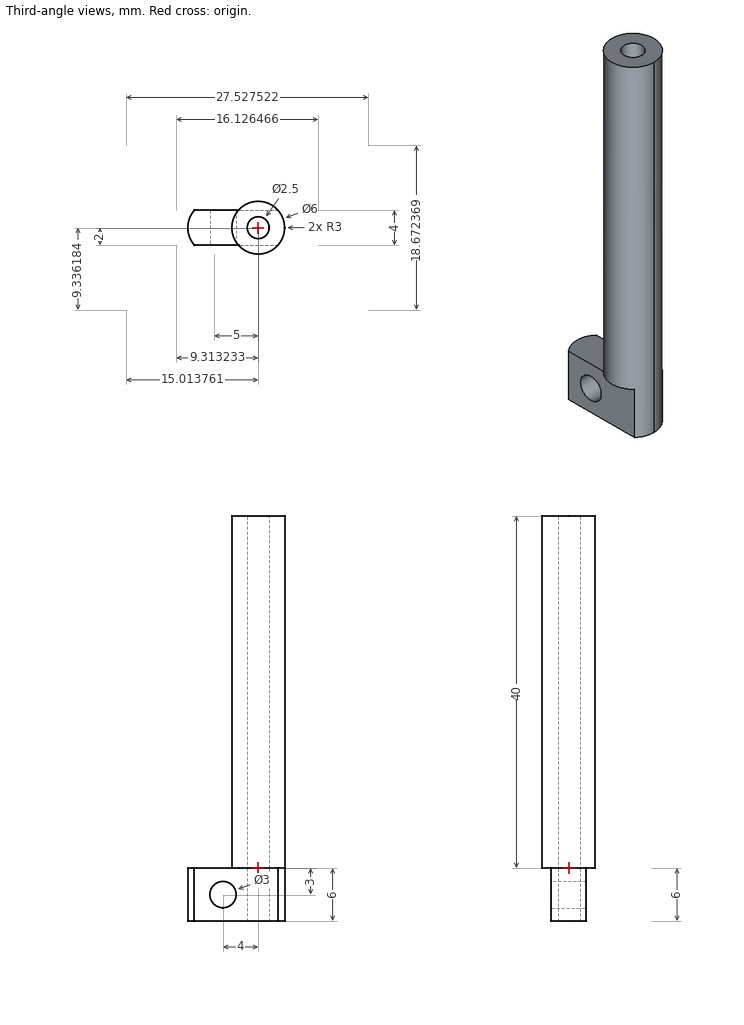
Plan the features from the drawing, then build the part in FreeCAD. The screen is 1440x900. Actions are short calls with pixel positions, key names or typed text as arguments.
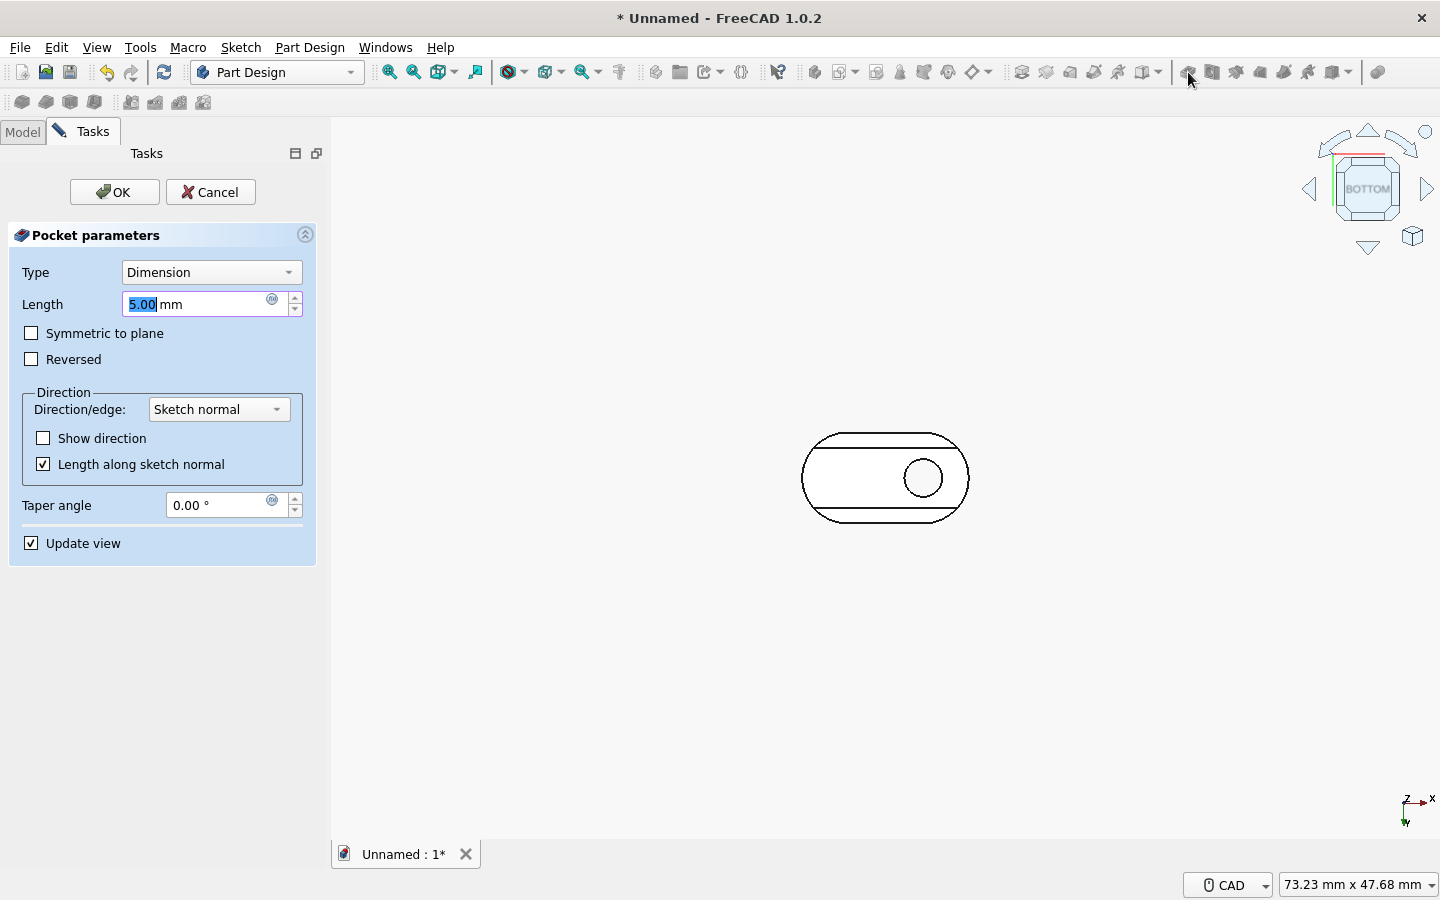
text(6)
key(Tab)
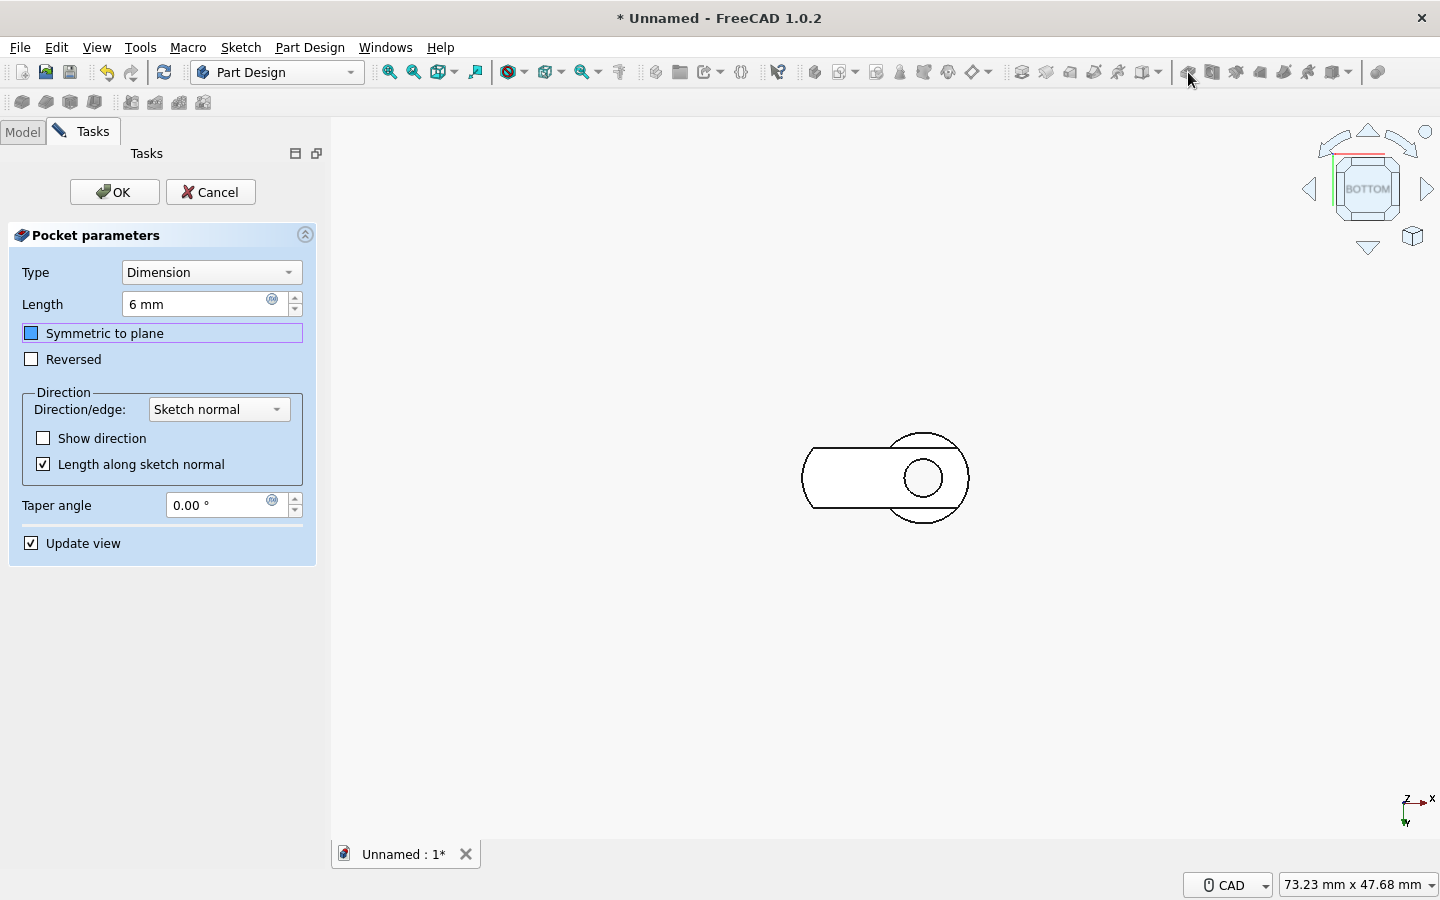
click(115, 192)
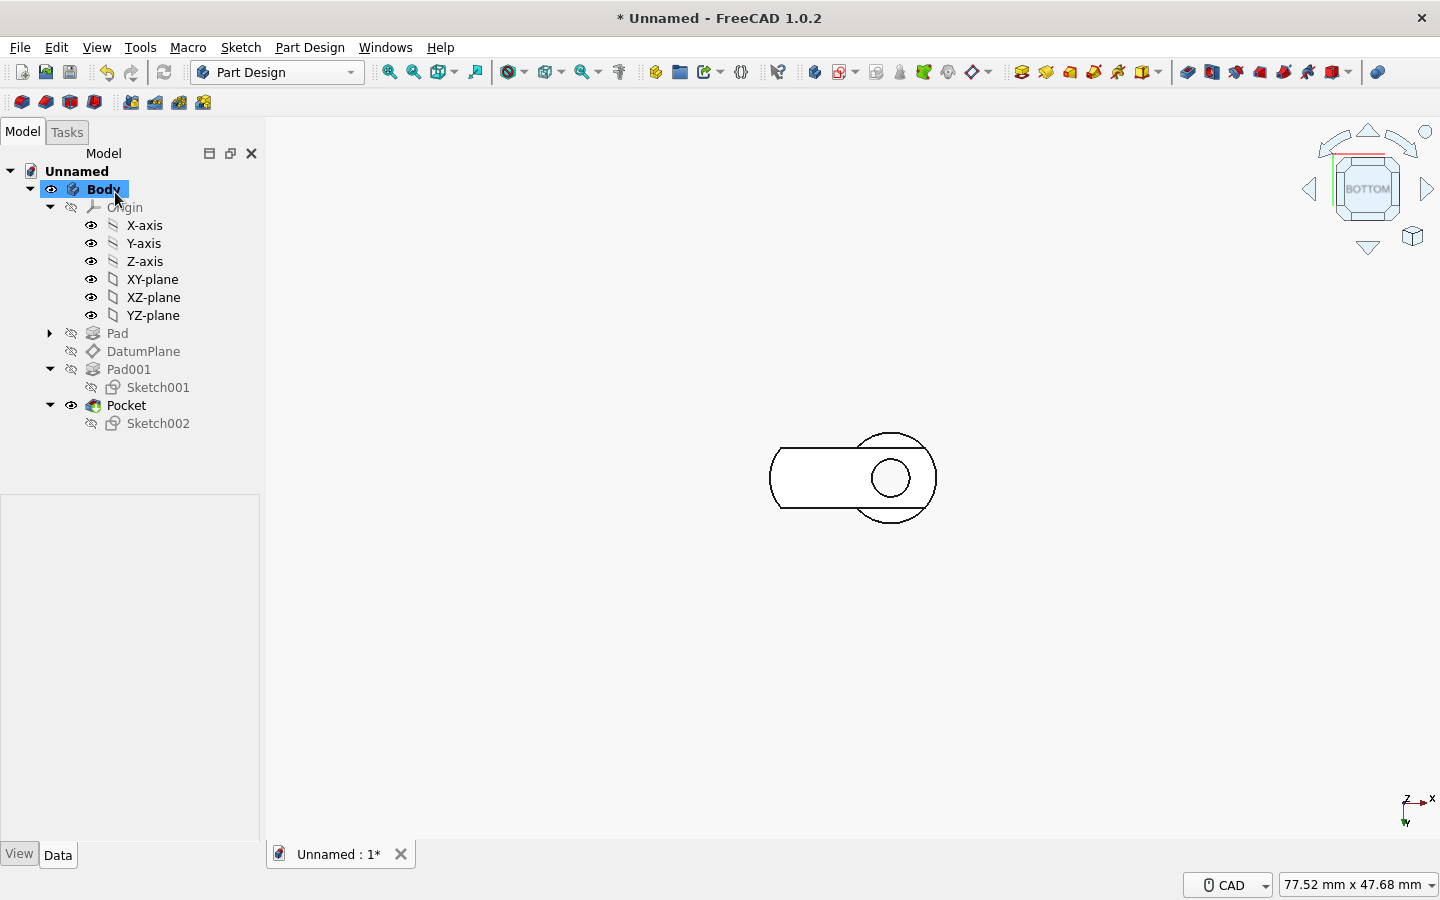
click(390, 72)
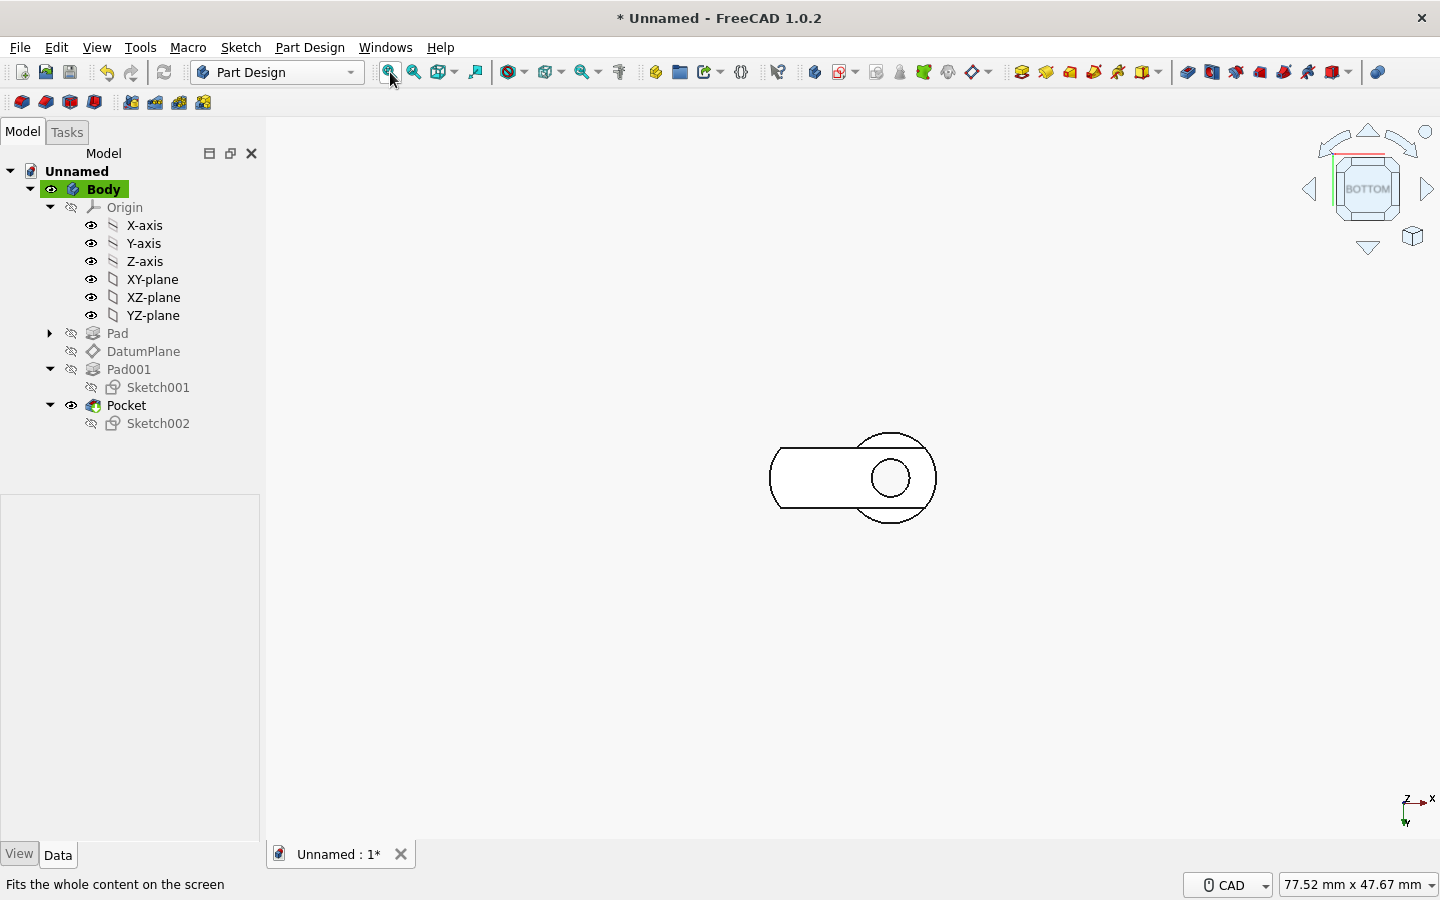
key(0)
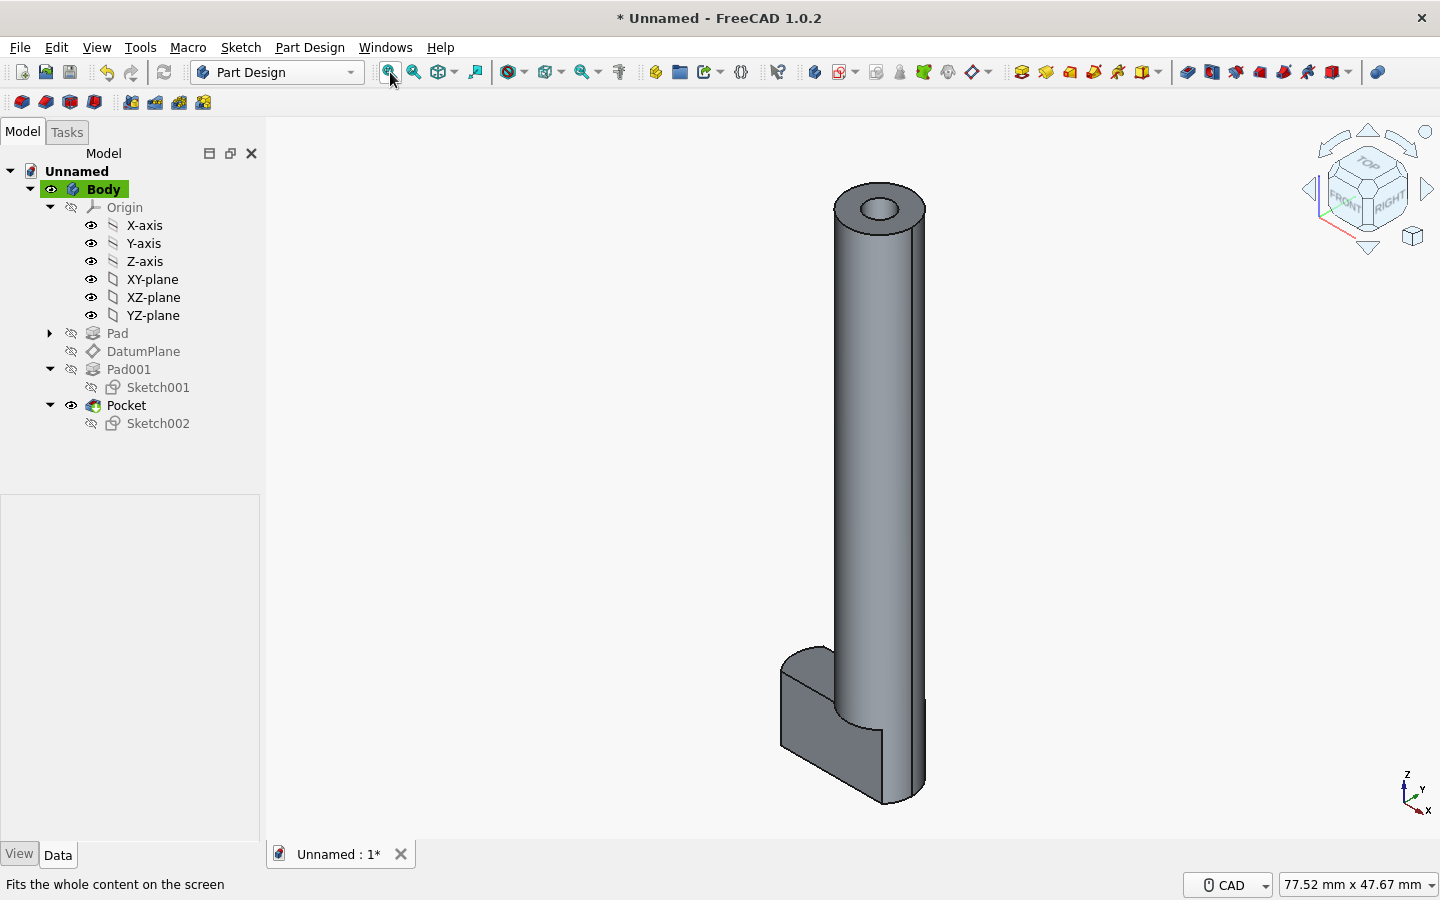
click(846, 745)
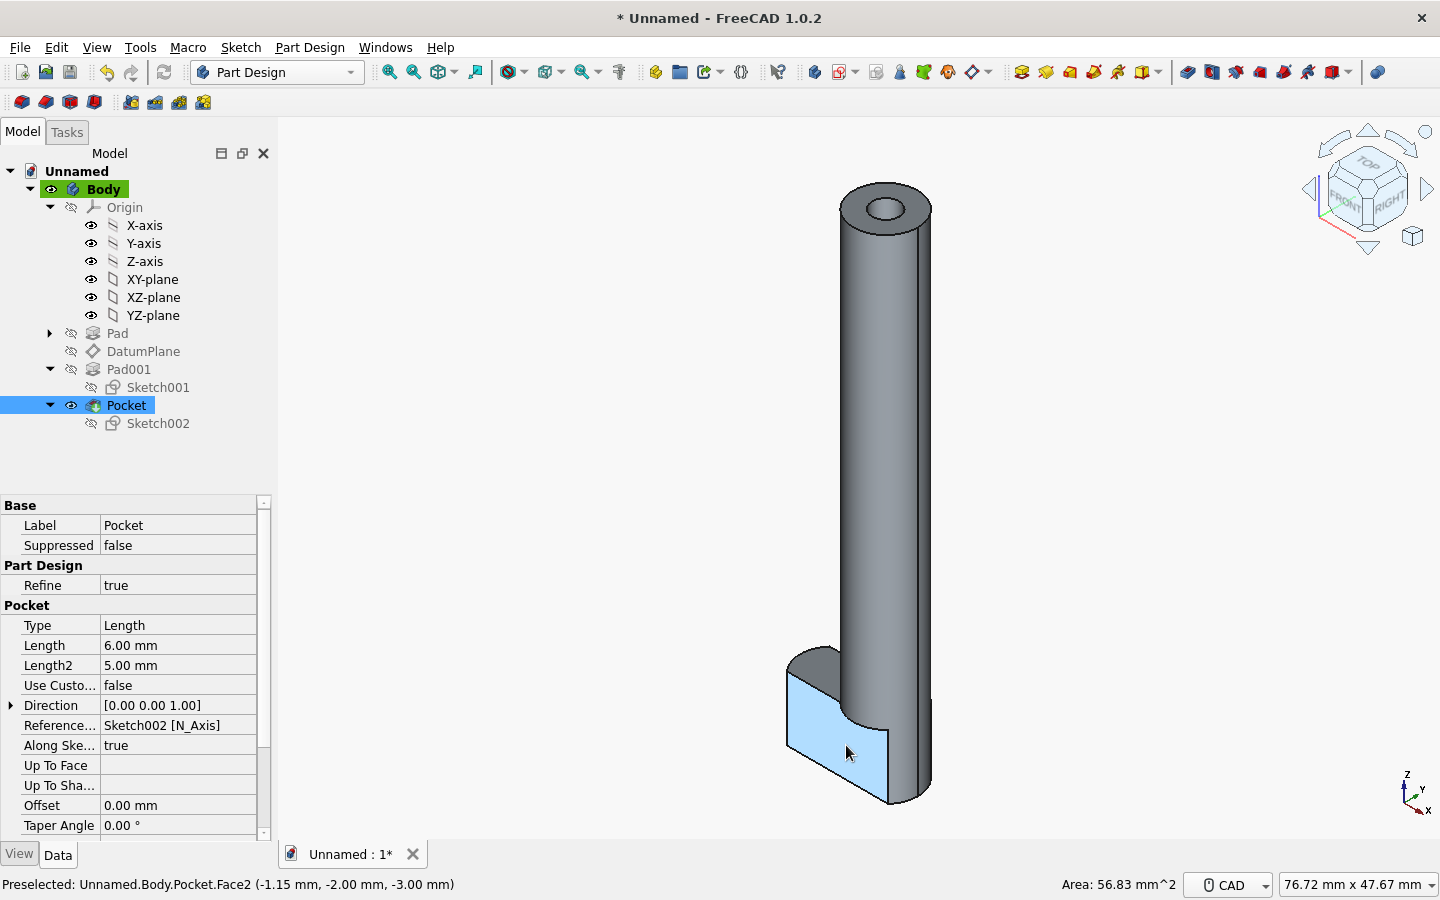
click(840, 72)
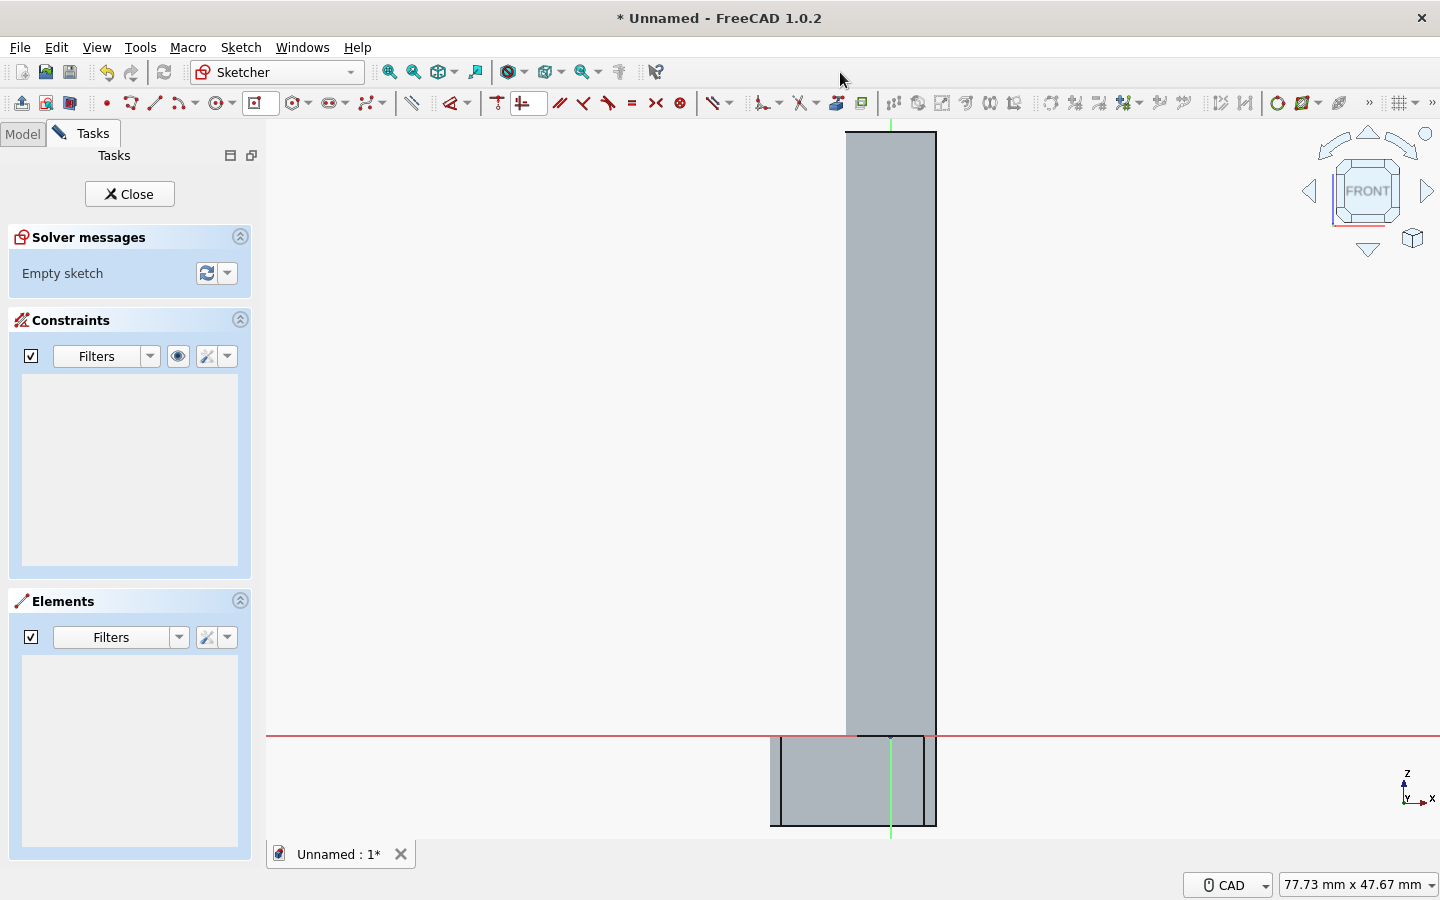
scroll(859, 811, up, 10)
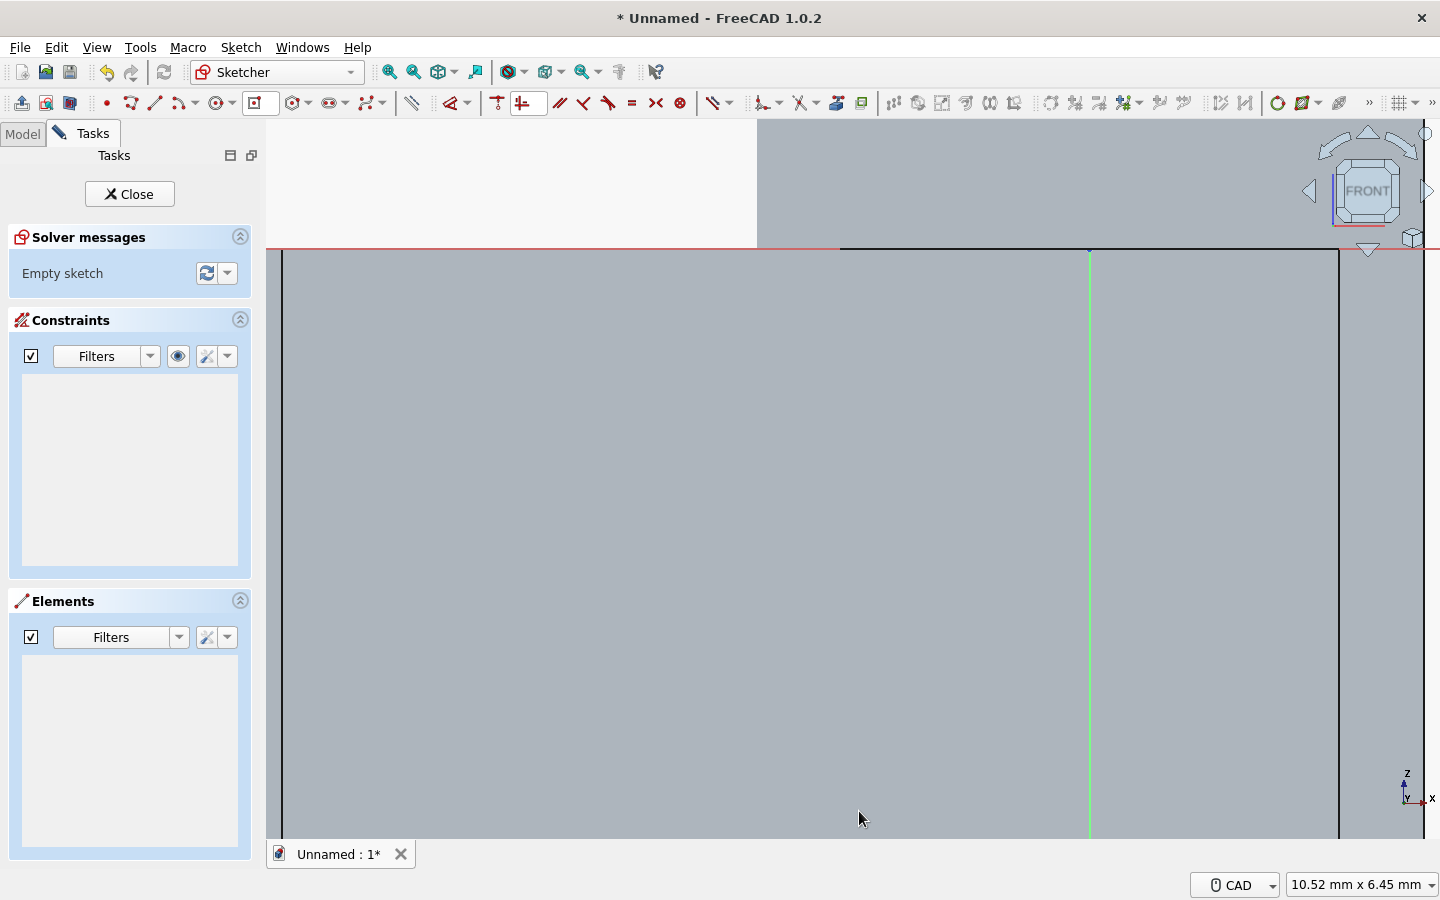
click(216, 104)